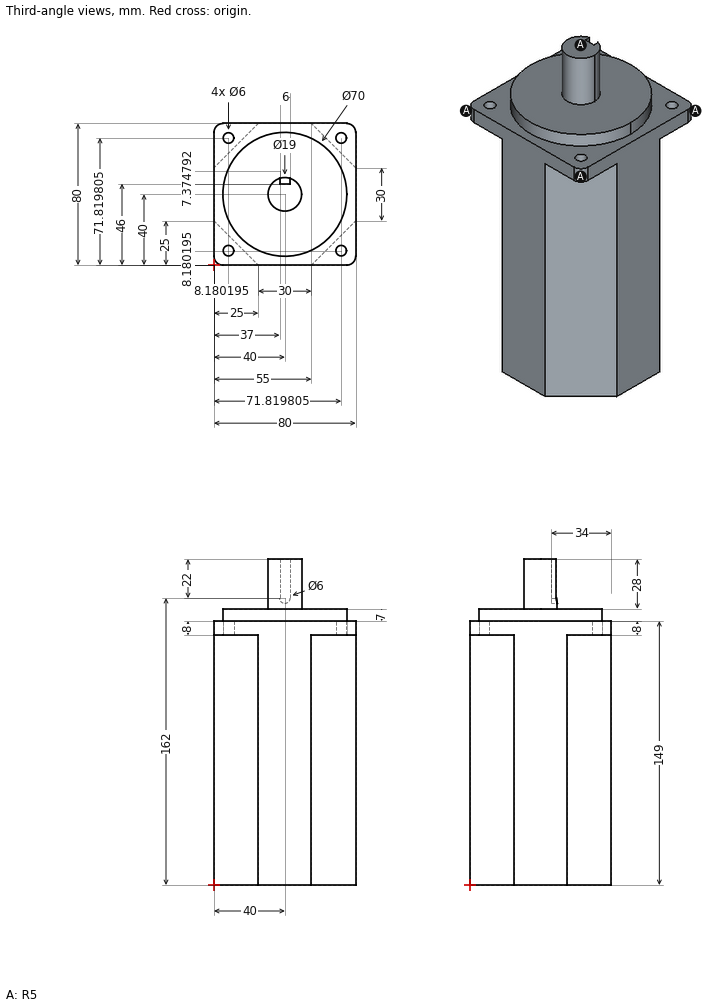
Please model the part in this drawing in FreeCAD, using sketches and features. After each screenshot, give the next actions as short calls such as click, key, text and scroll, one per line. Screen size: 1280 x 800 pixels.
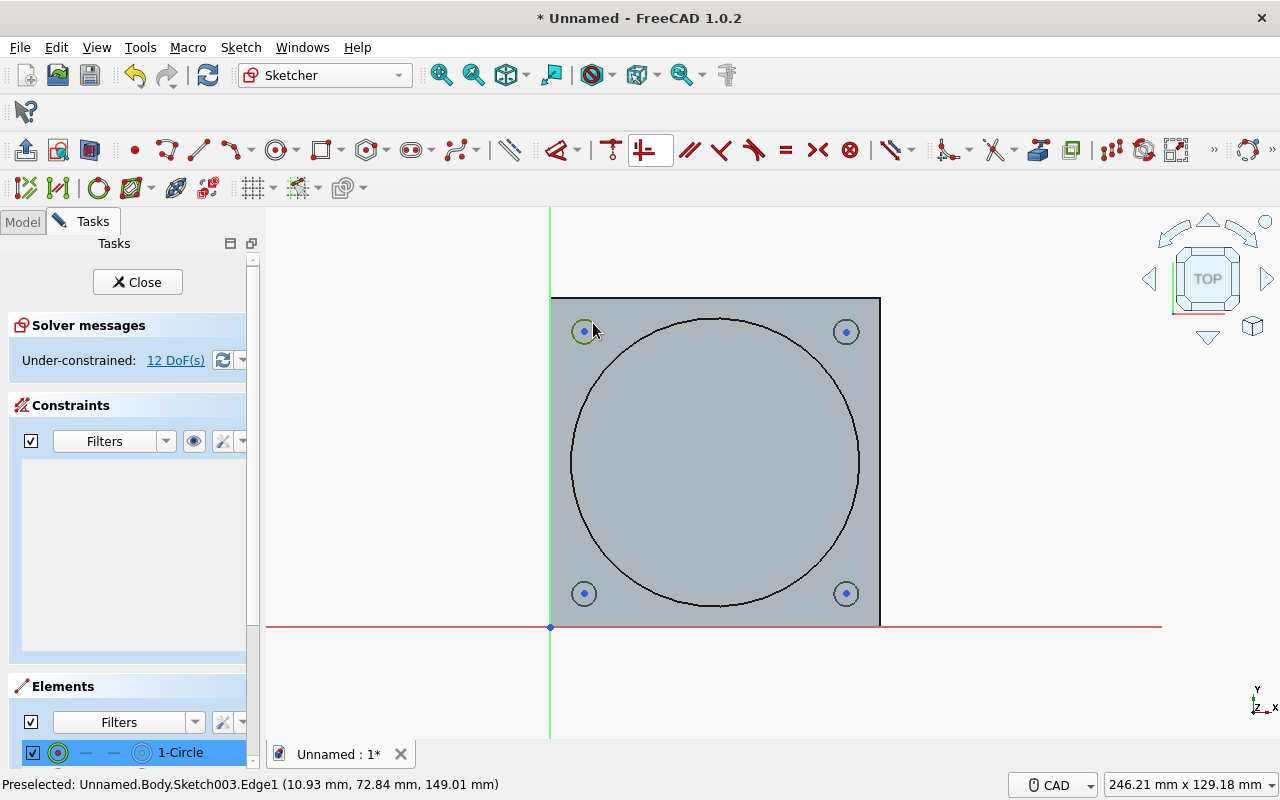
click(855, 323)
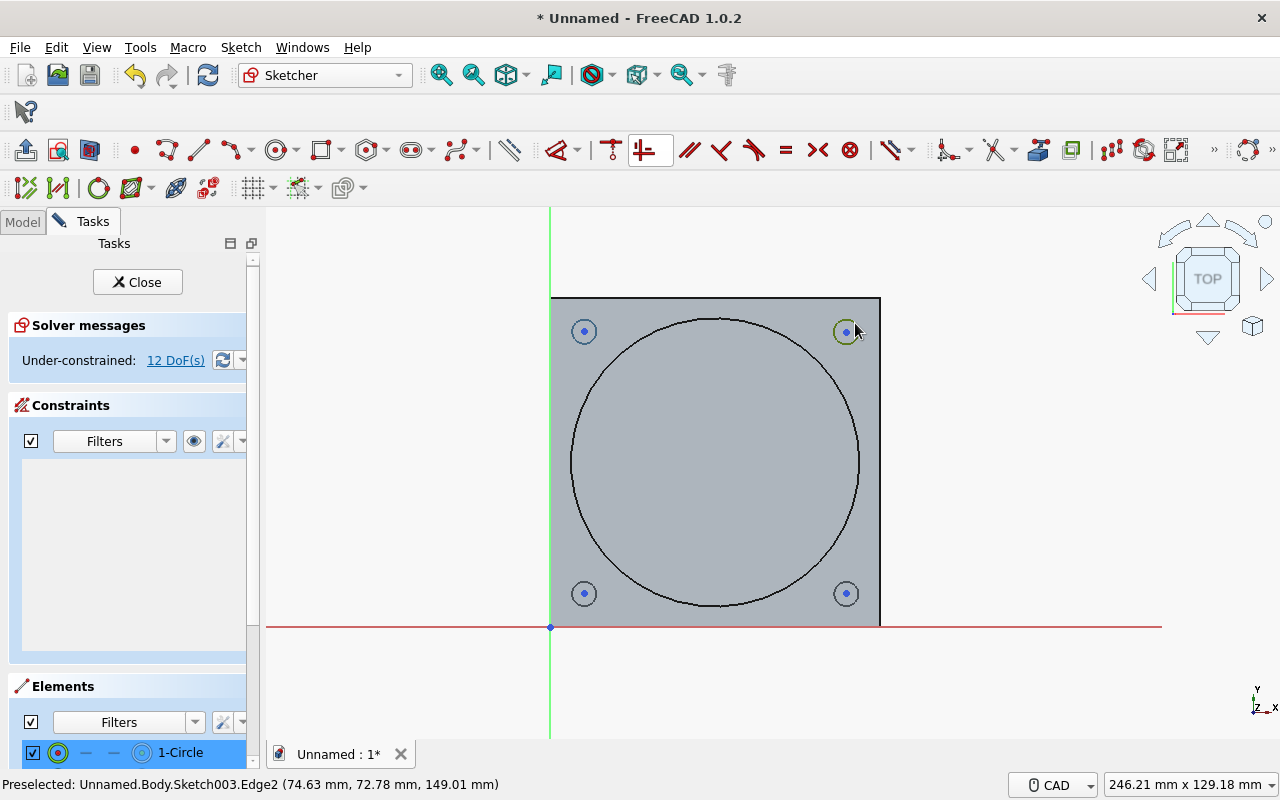
click(855, 585)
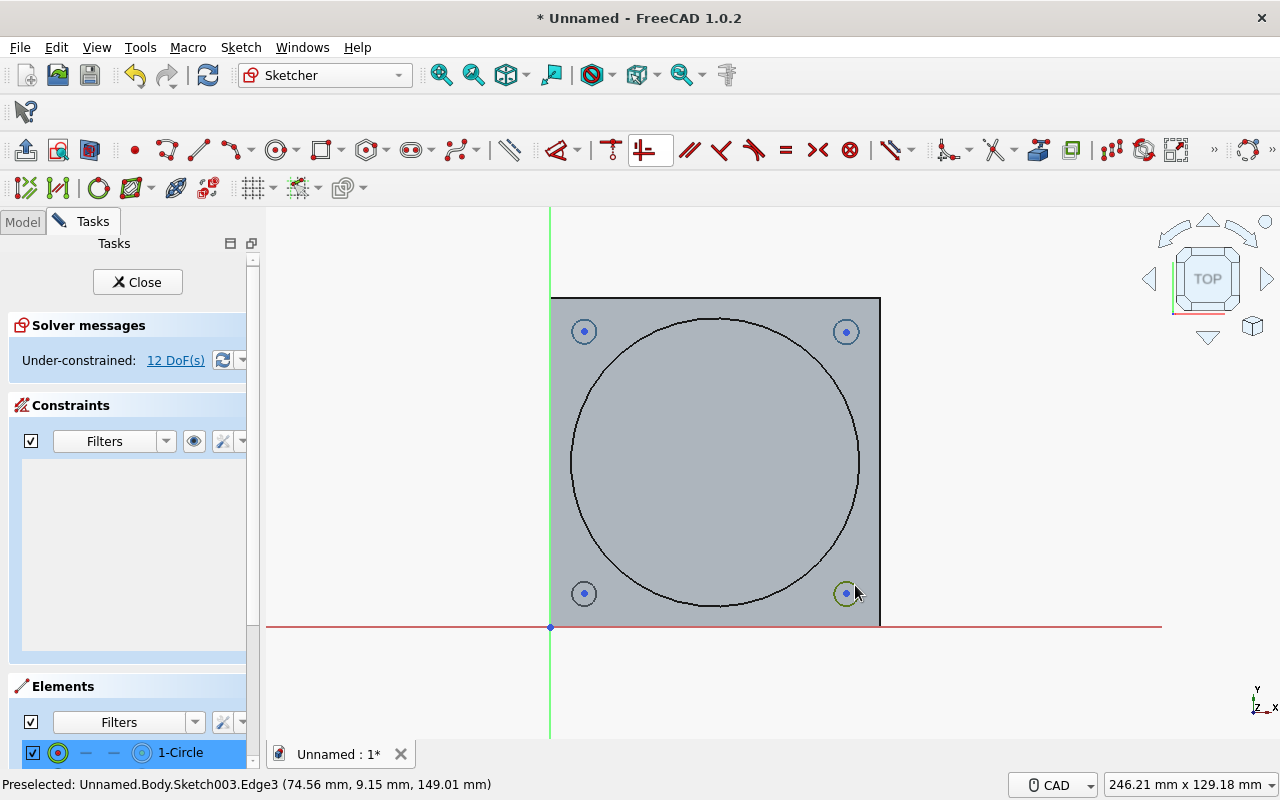
click(593, 585)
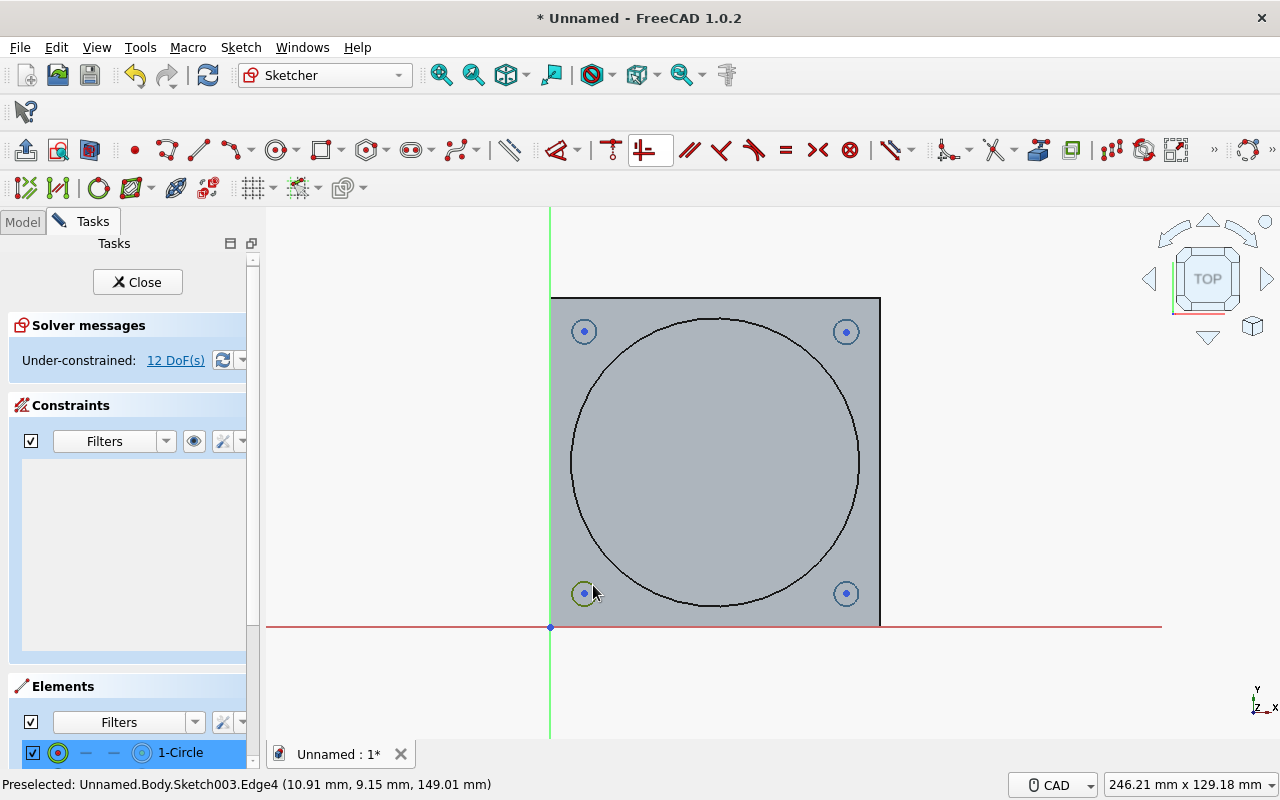
key(e)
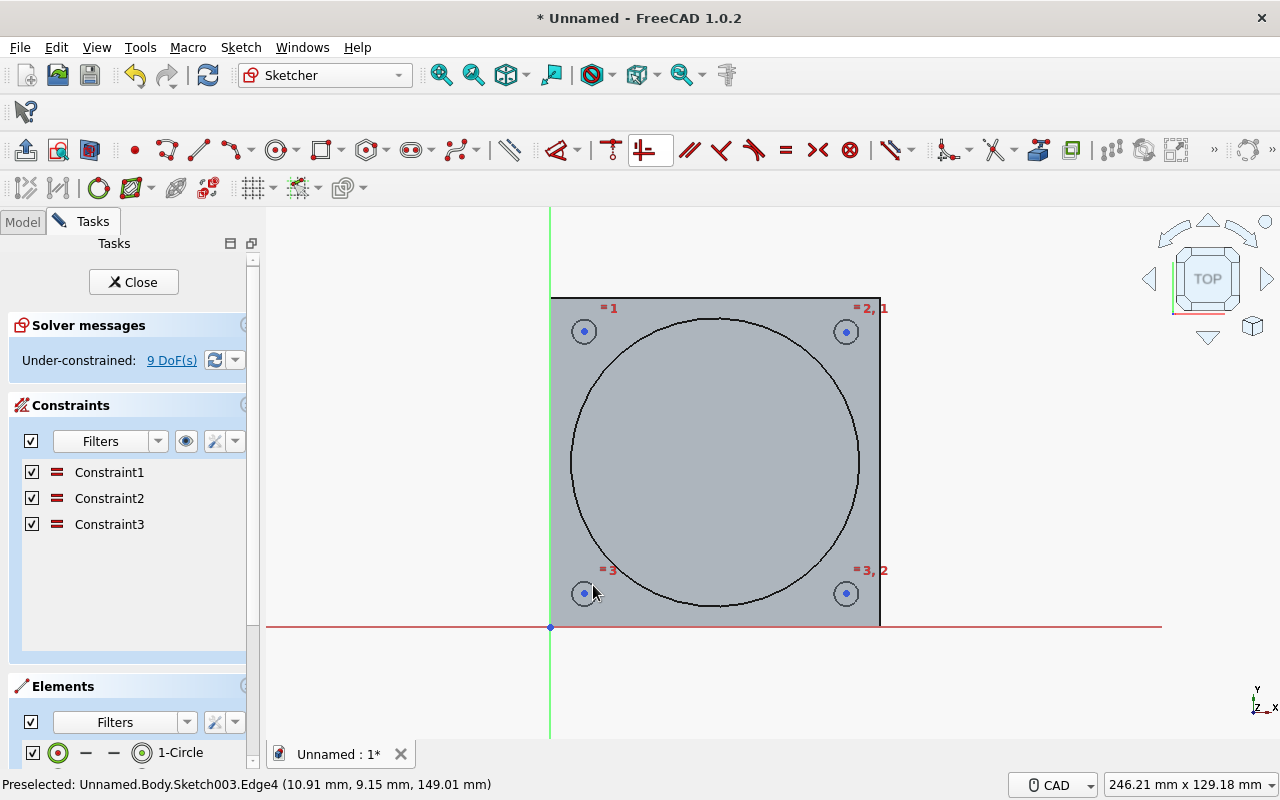
click(584, 332)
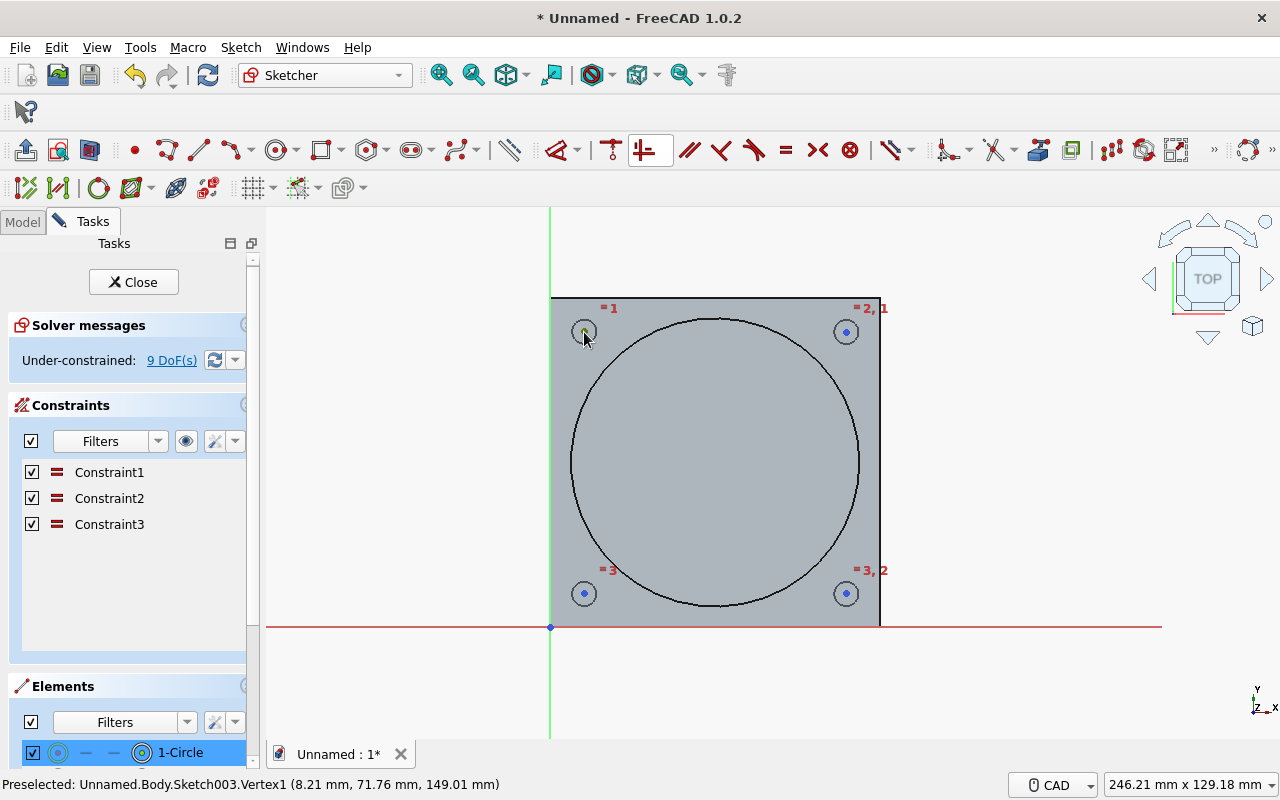
click(846, 332)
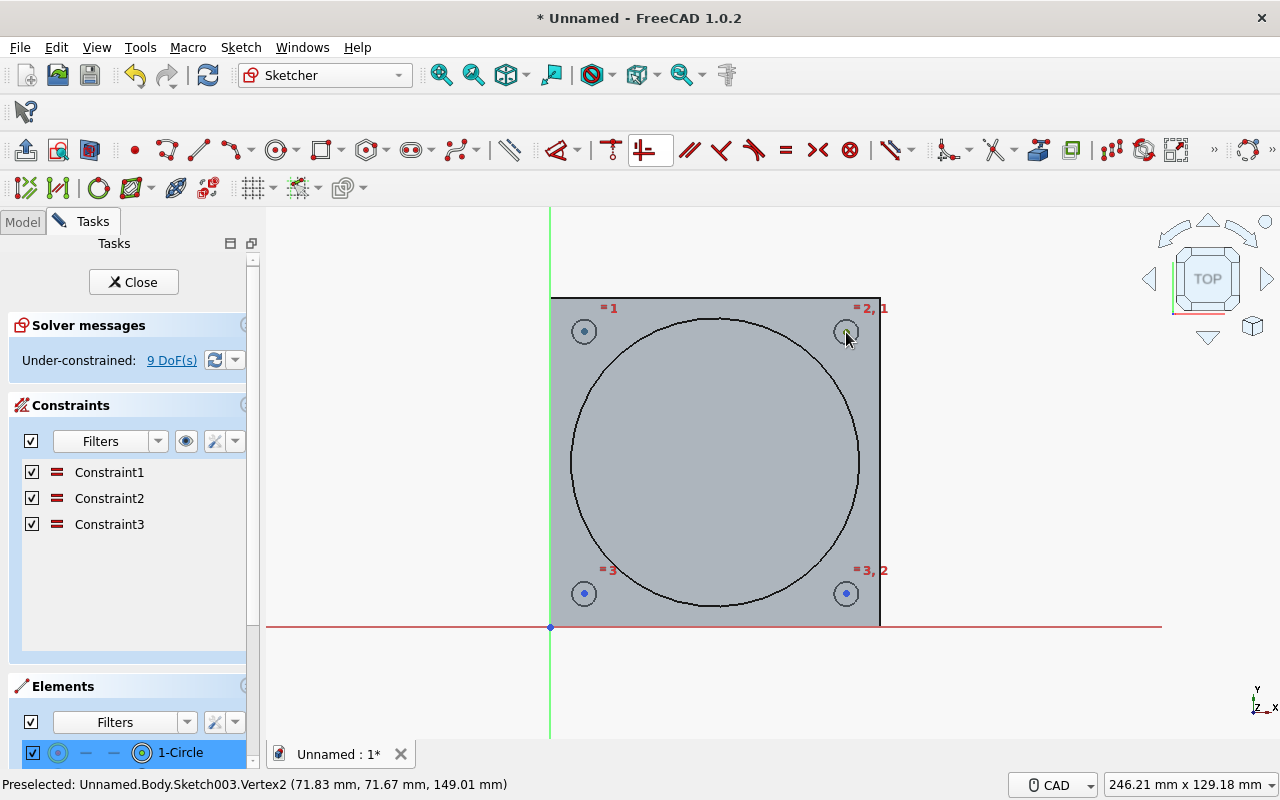
key(h)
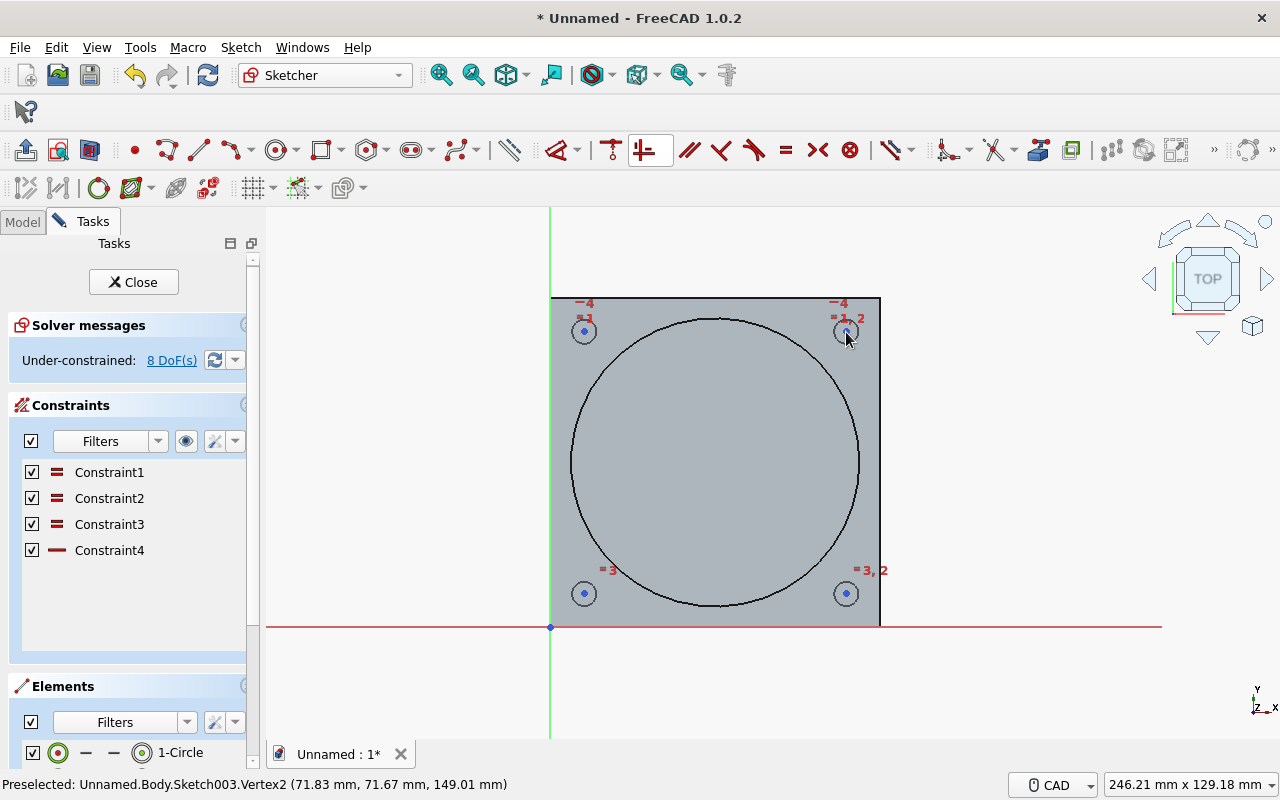
click(846, 332)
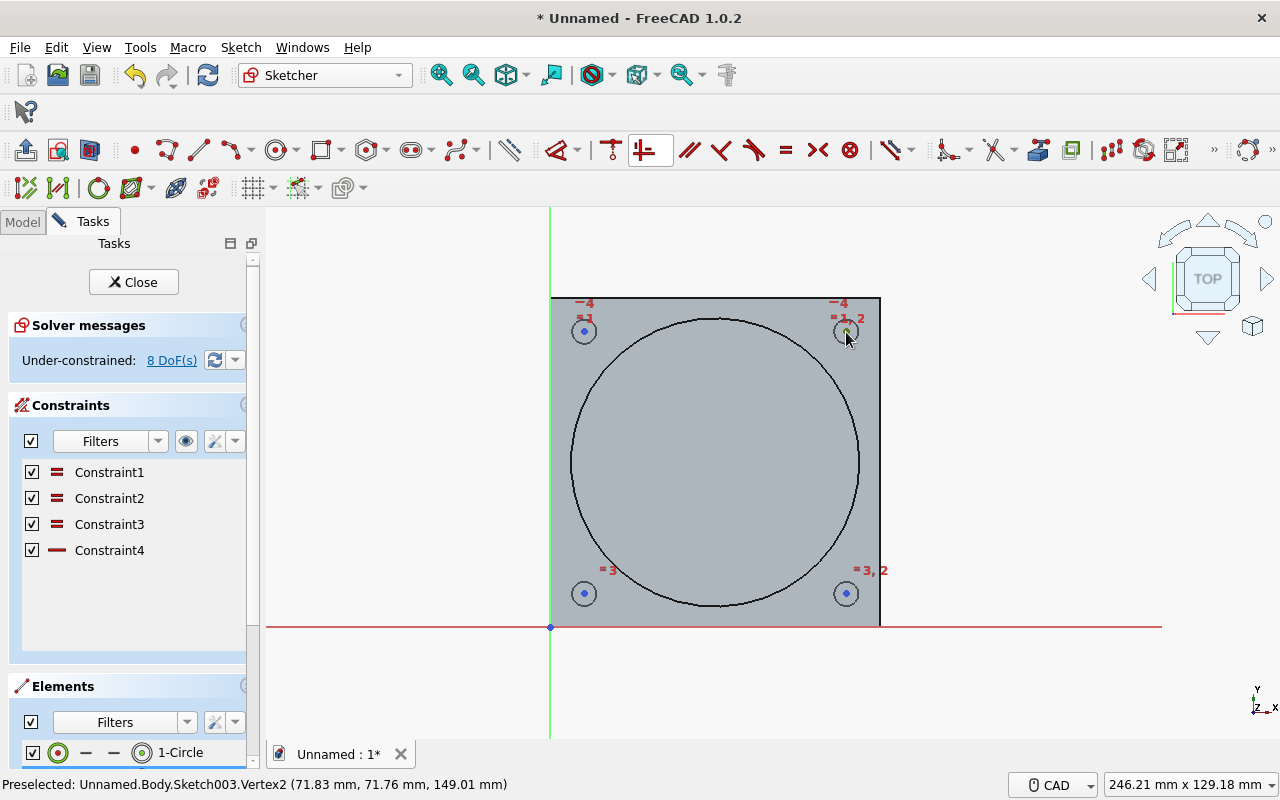
click(846, 594)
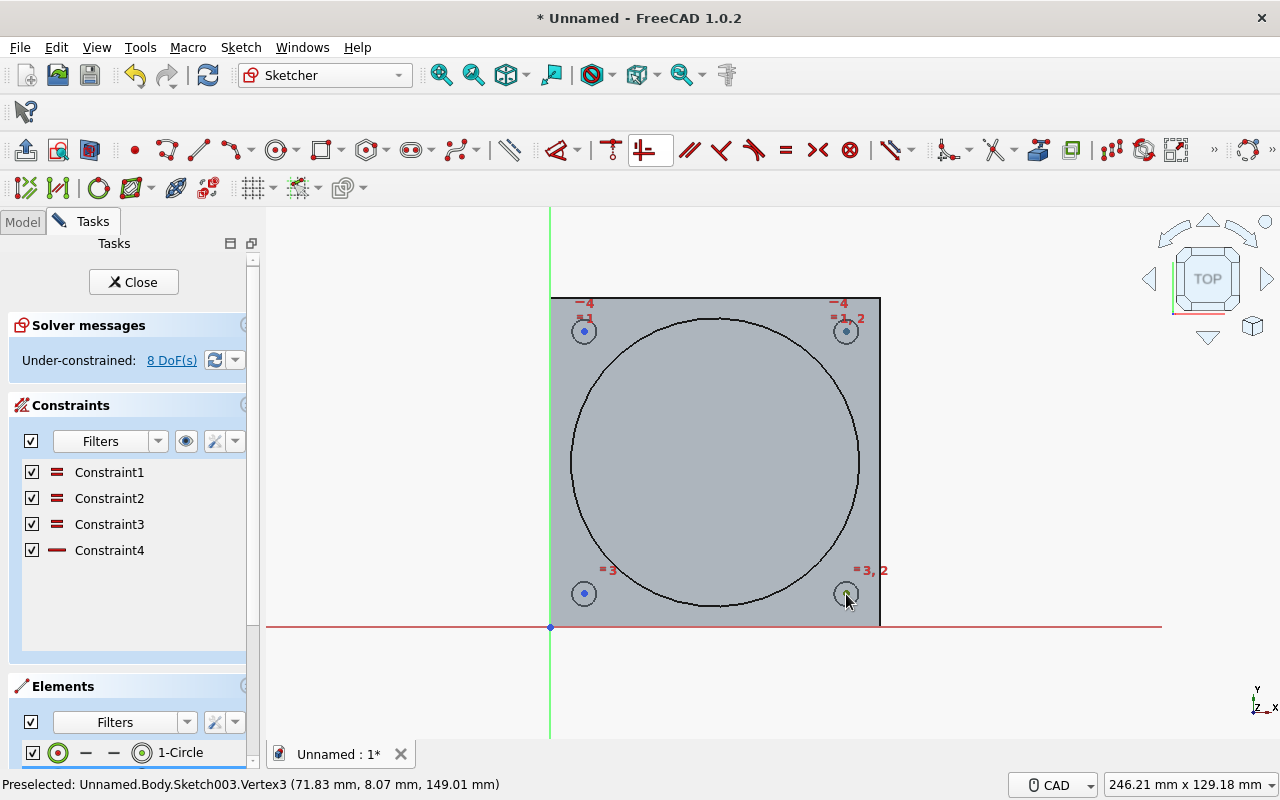
key(v)